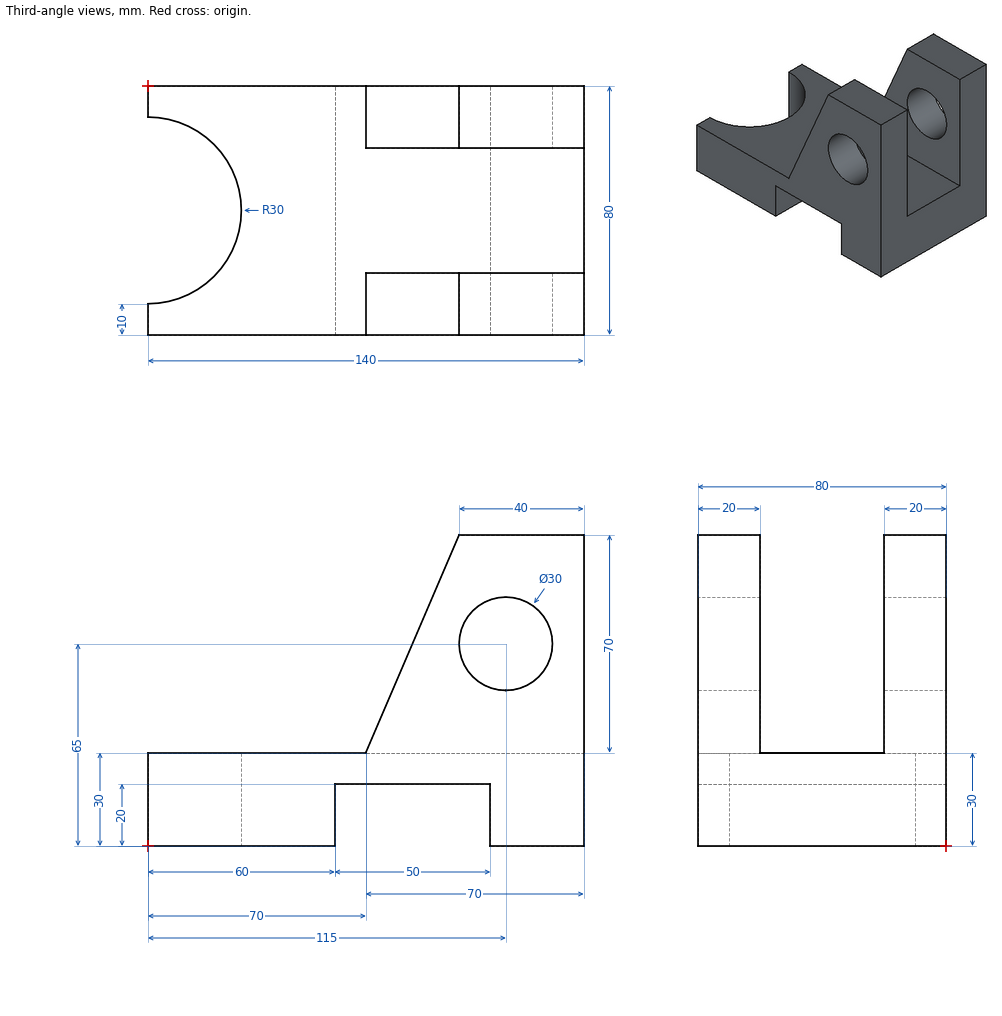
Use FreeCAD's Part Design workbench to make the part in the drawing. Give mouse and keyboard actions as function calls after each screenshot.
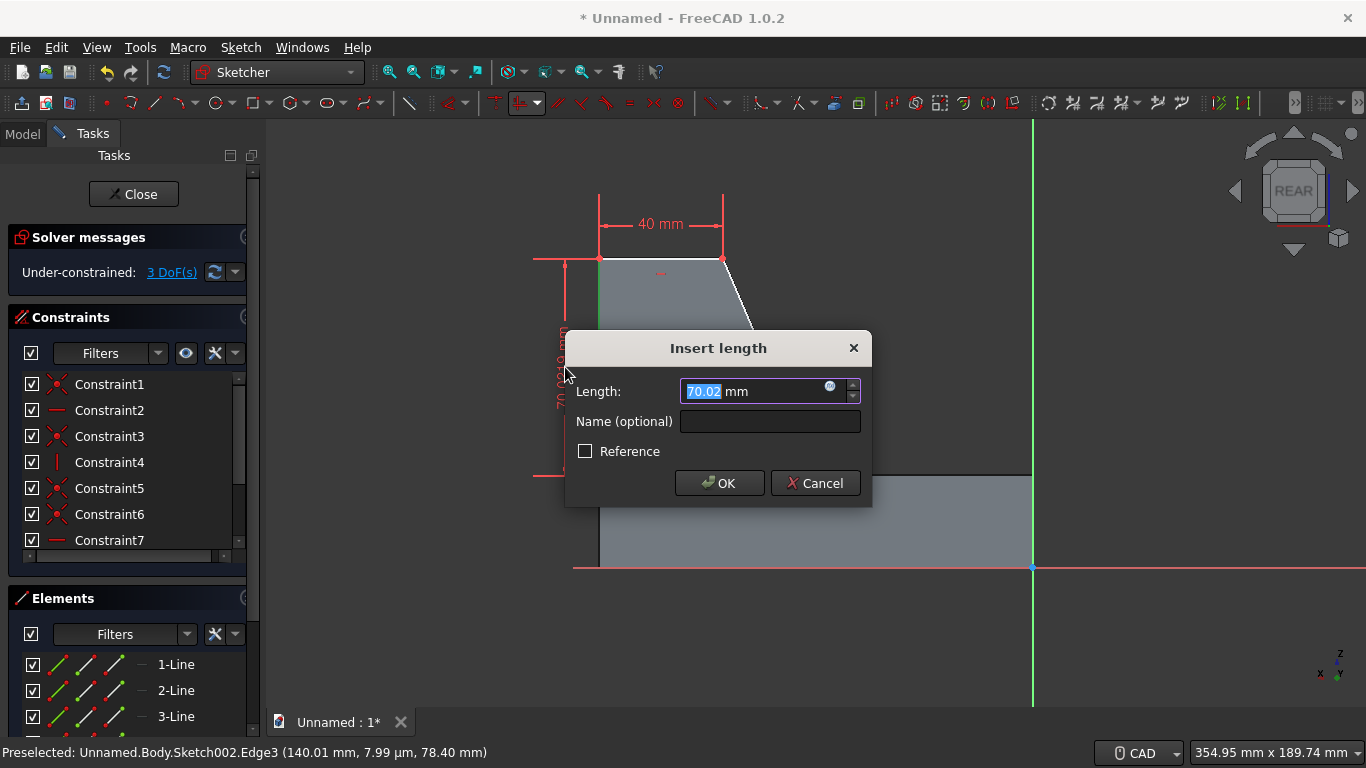
text(70)
key(Return)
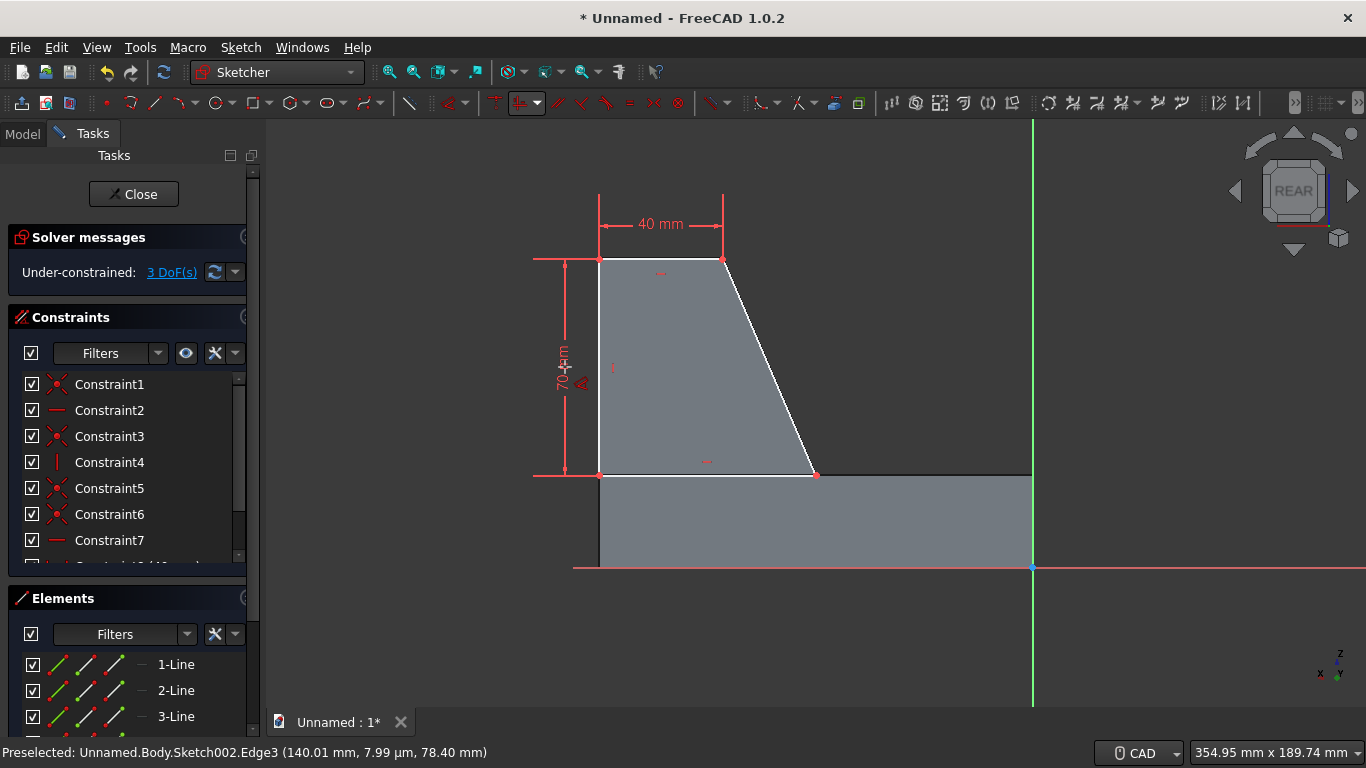
click(664, 476)
click(708, 510)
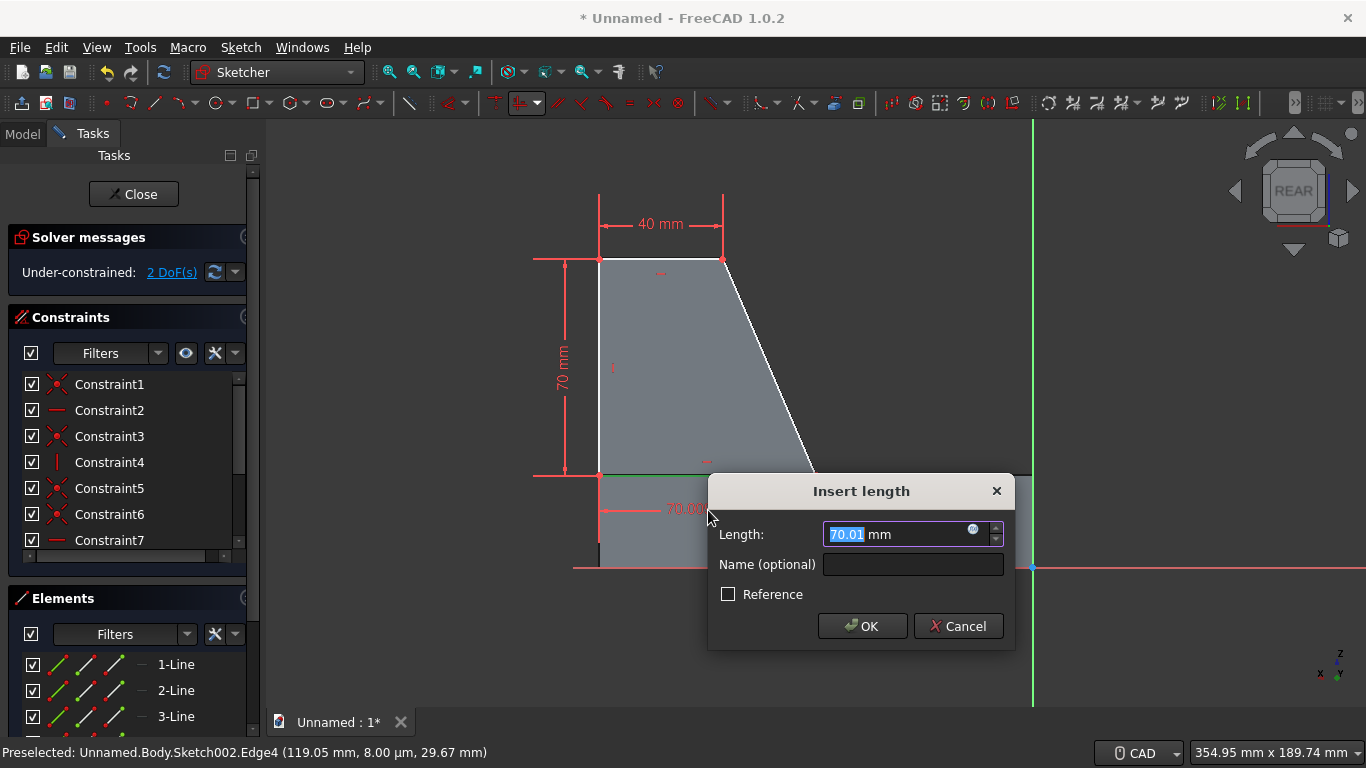
text(70)
key(Return)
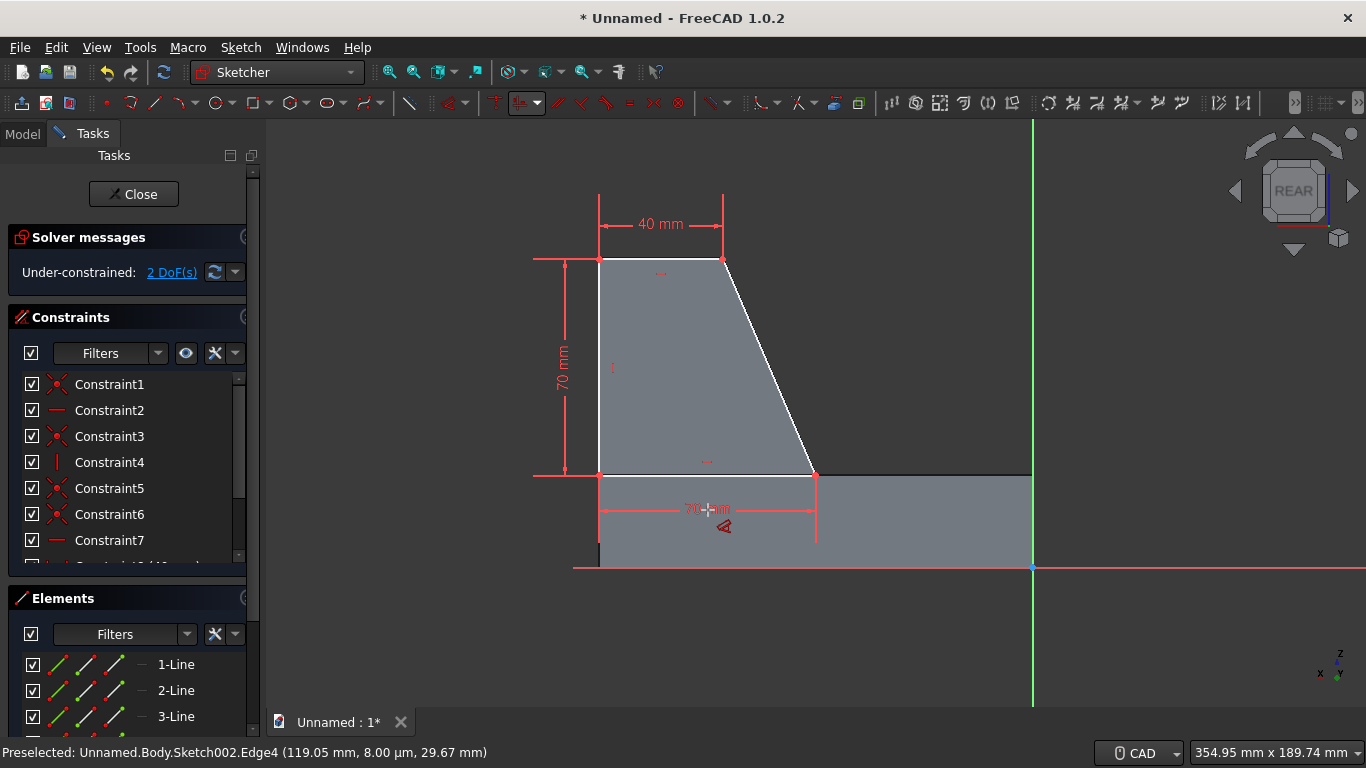
click(816, 476)
click(924, 602)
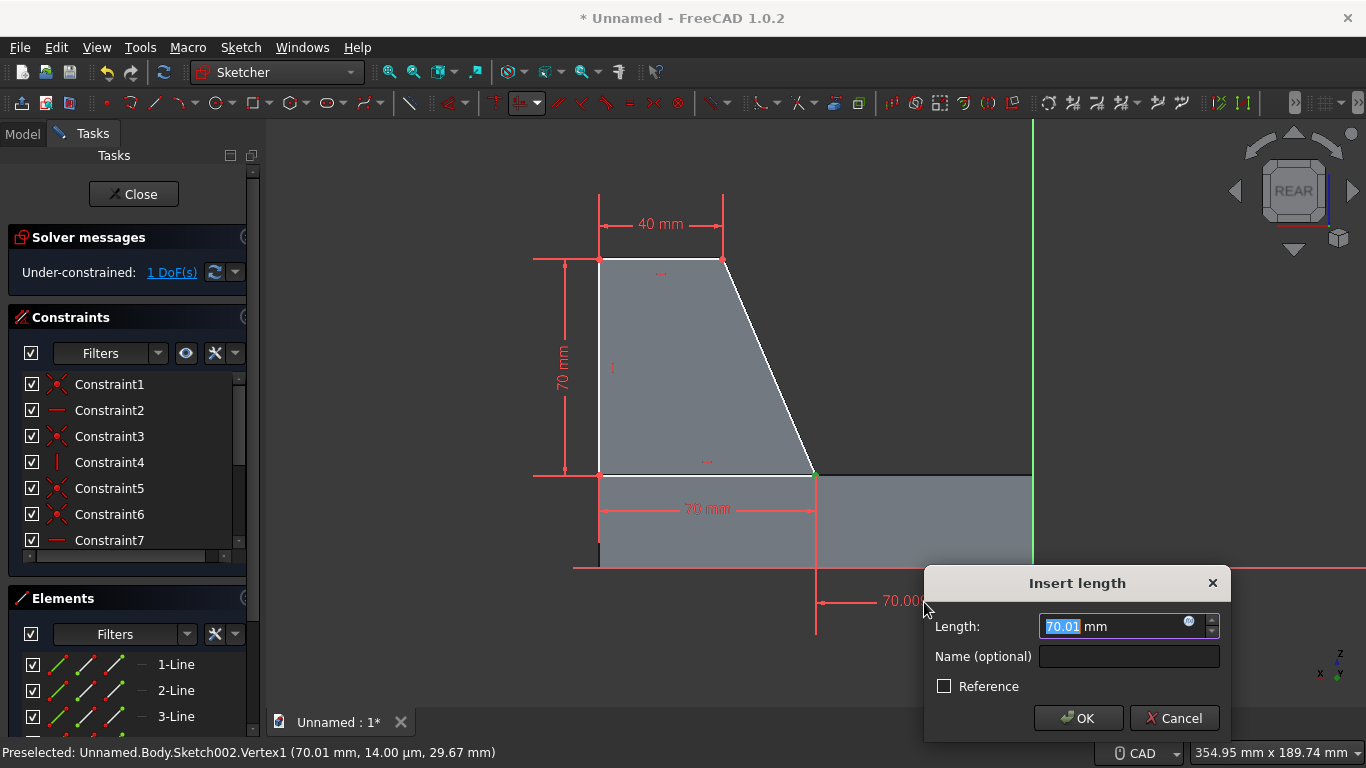
text(70)
key(Return)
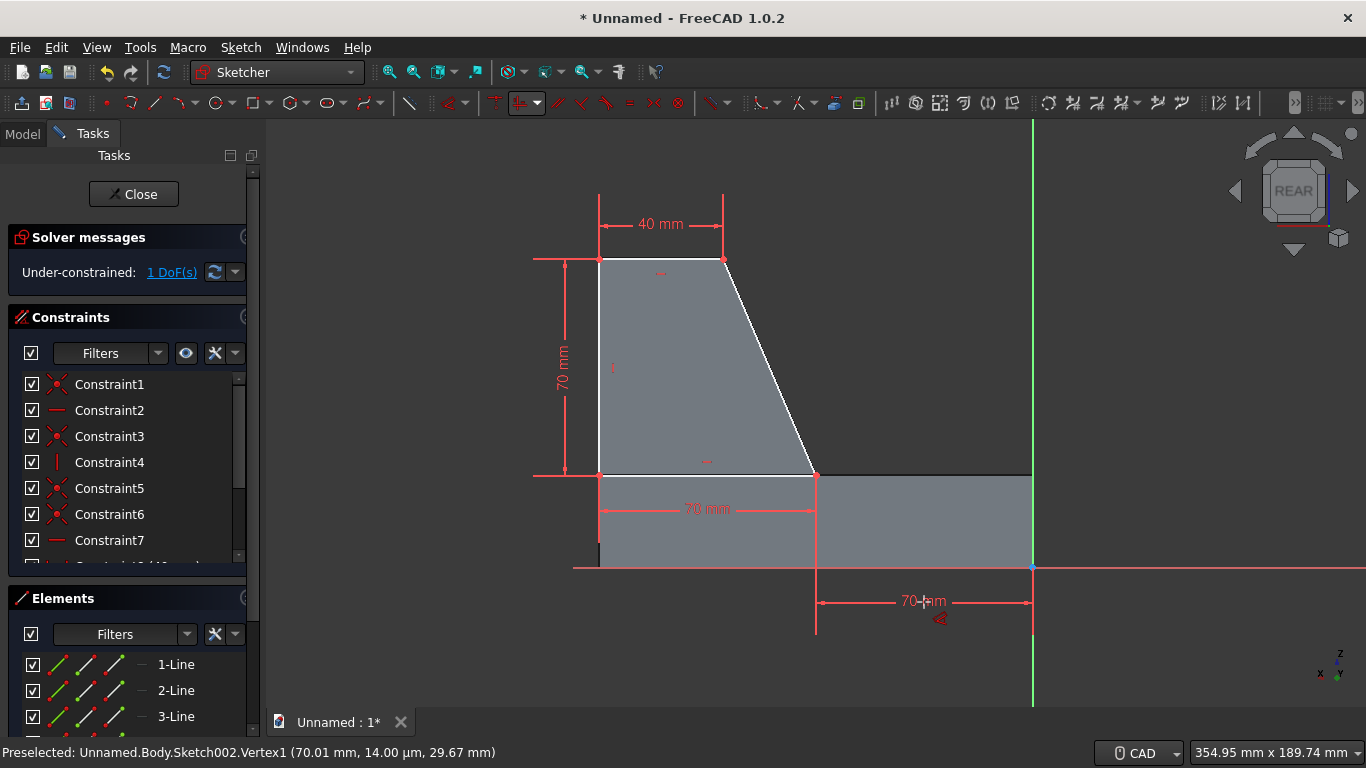
click(816, 476)
click(1067, 522)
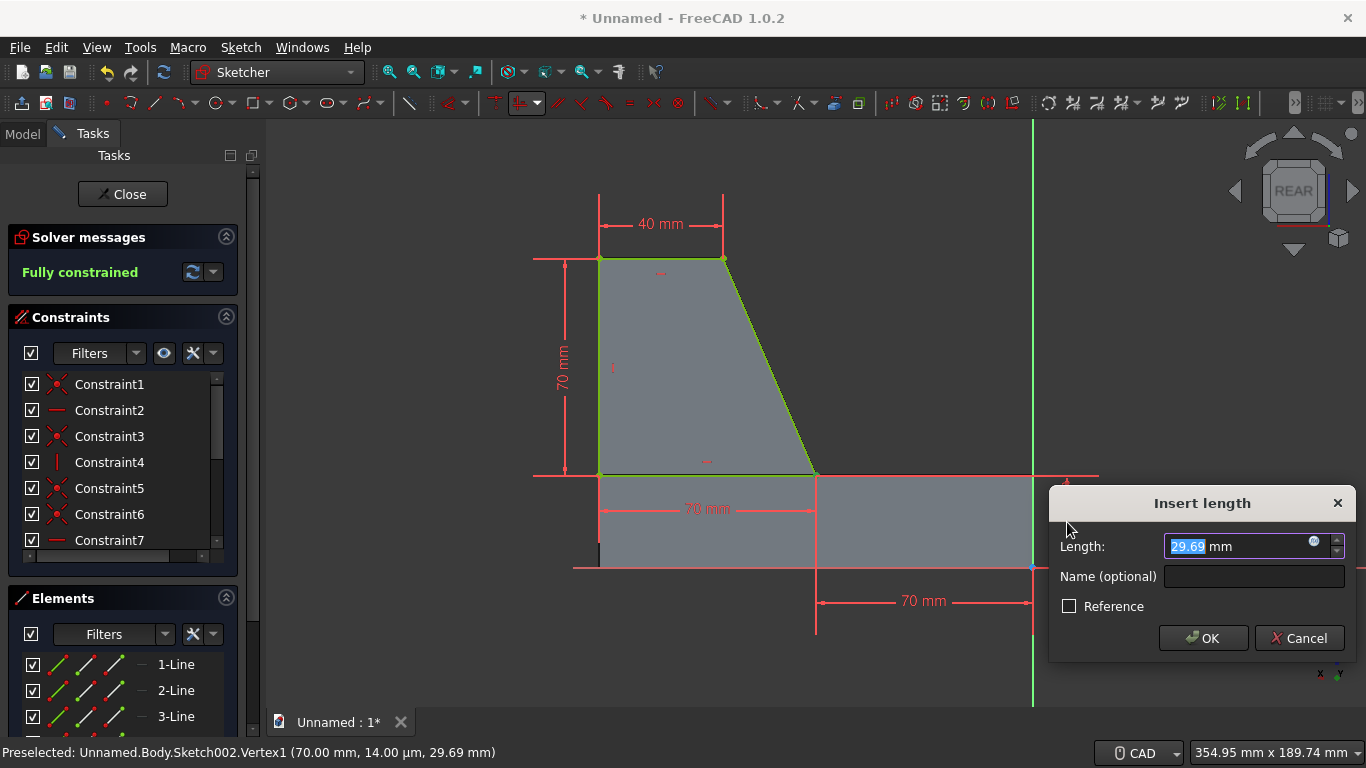
text(30)
key(Return)
key(Escape)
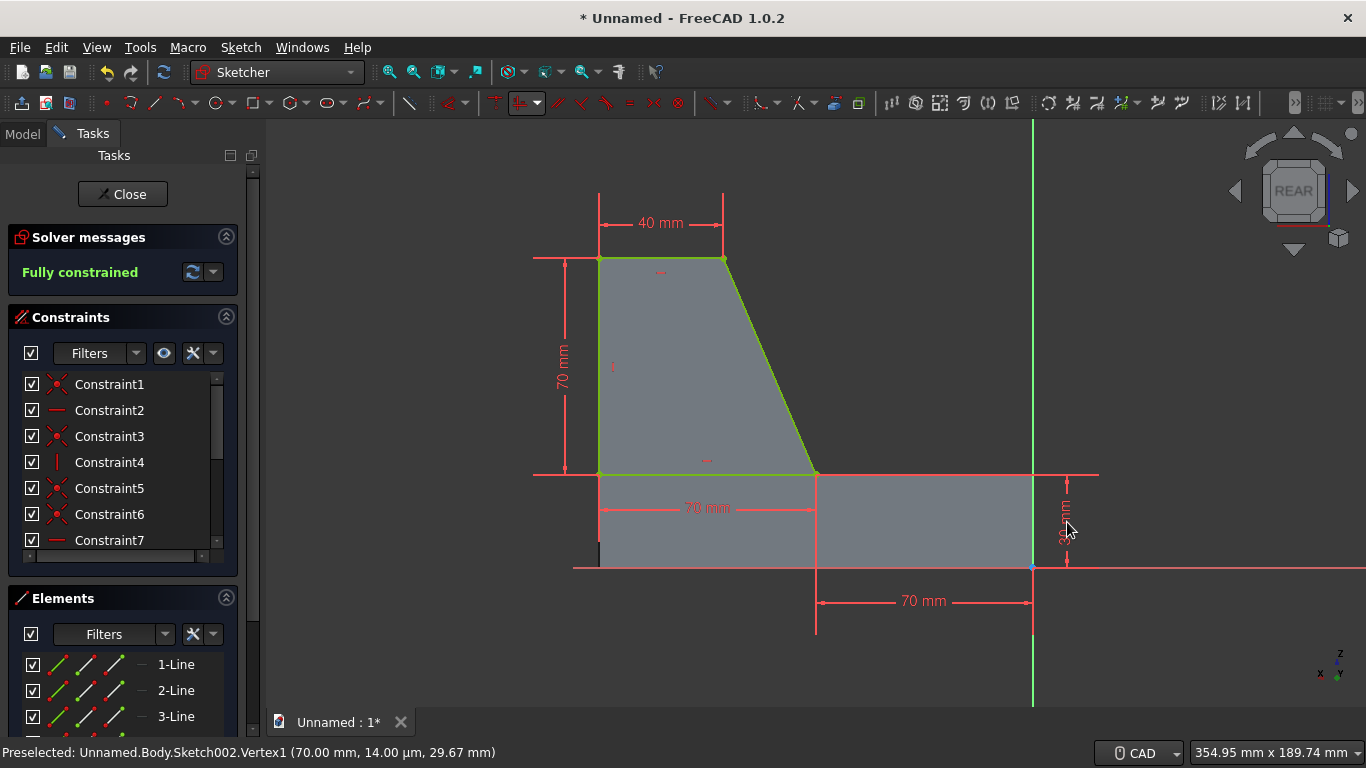
click(123, 194)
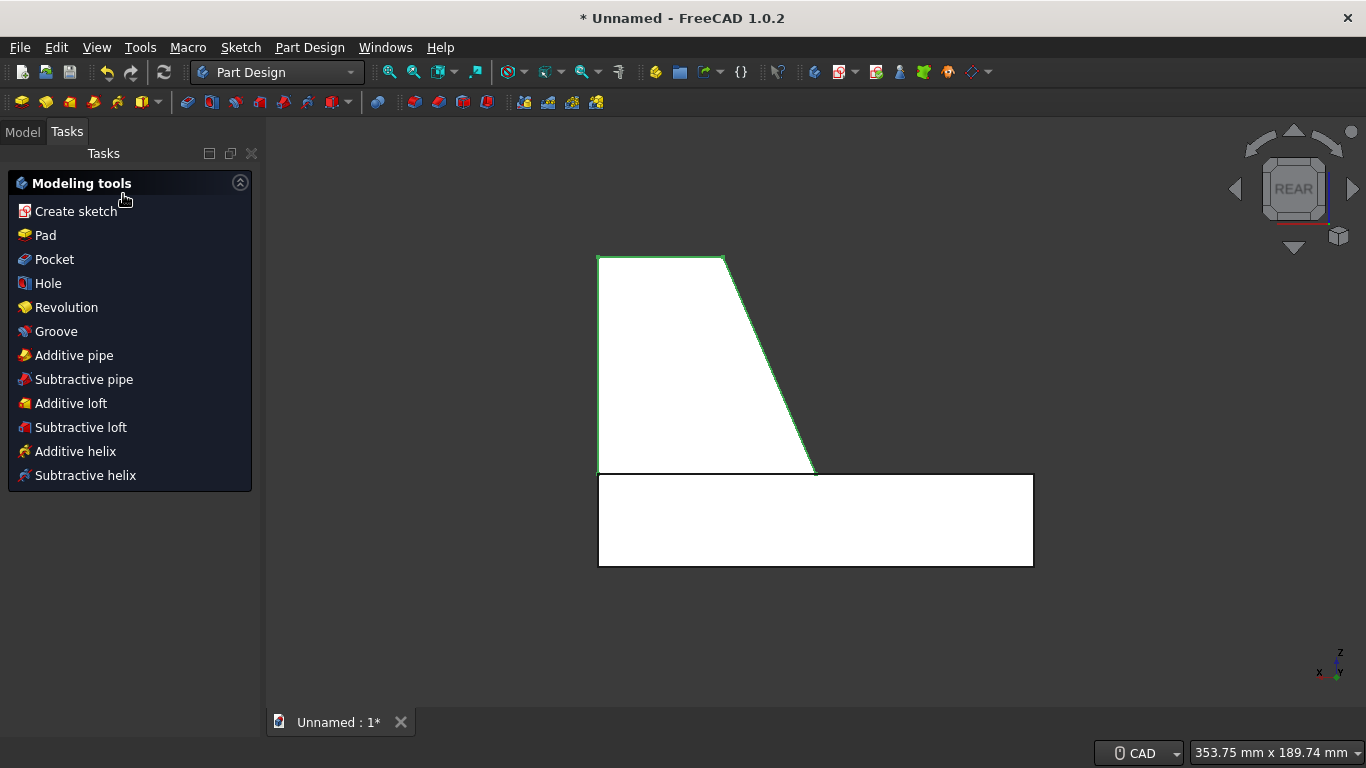
click(22, 102)